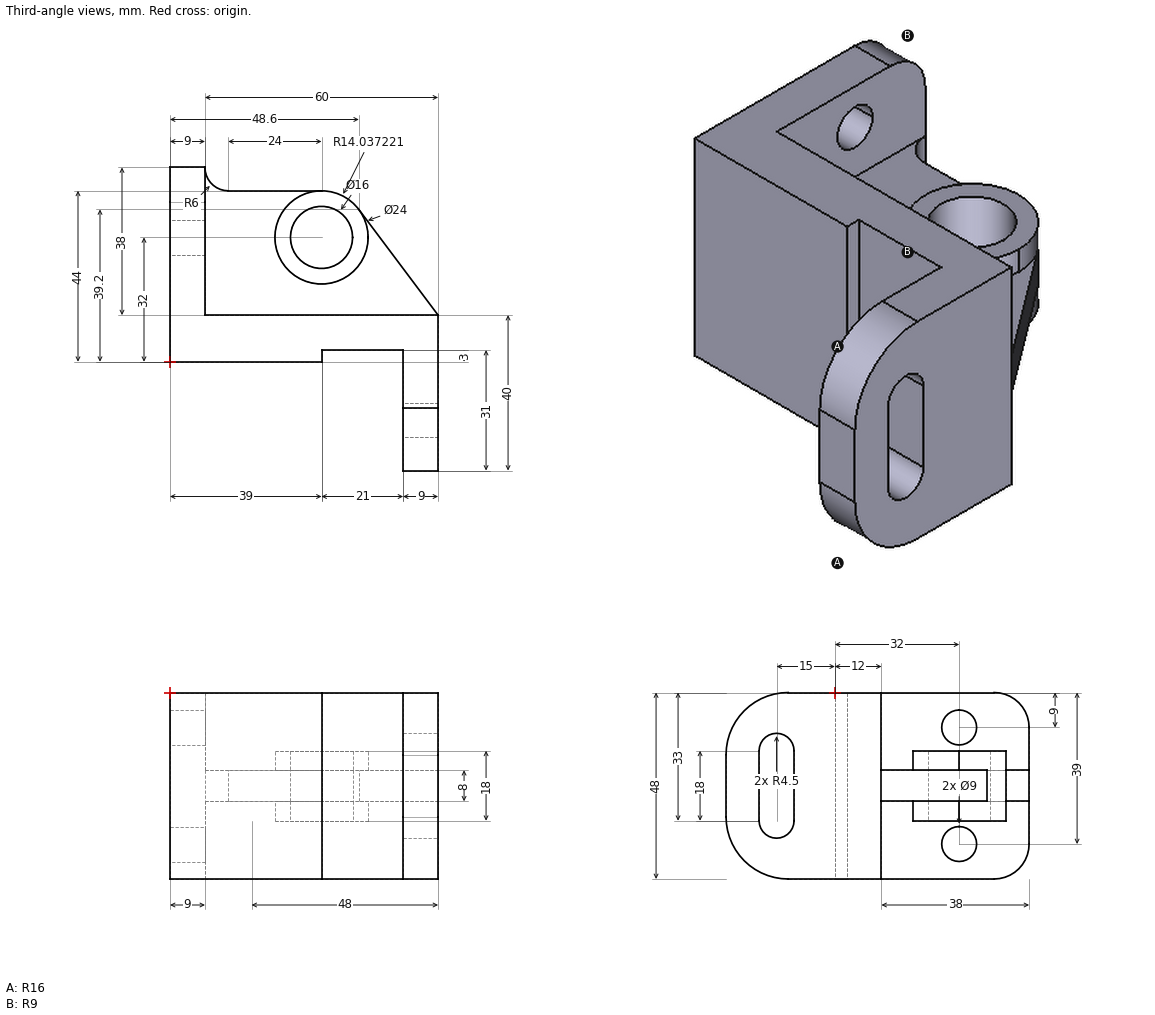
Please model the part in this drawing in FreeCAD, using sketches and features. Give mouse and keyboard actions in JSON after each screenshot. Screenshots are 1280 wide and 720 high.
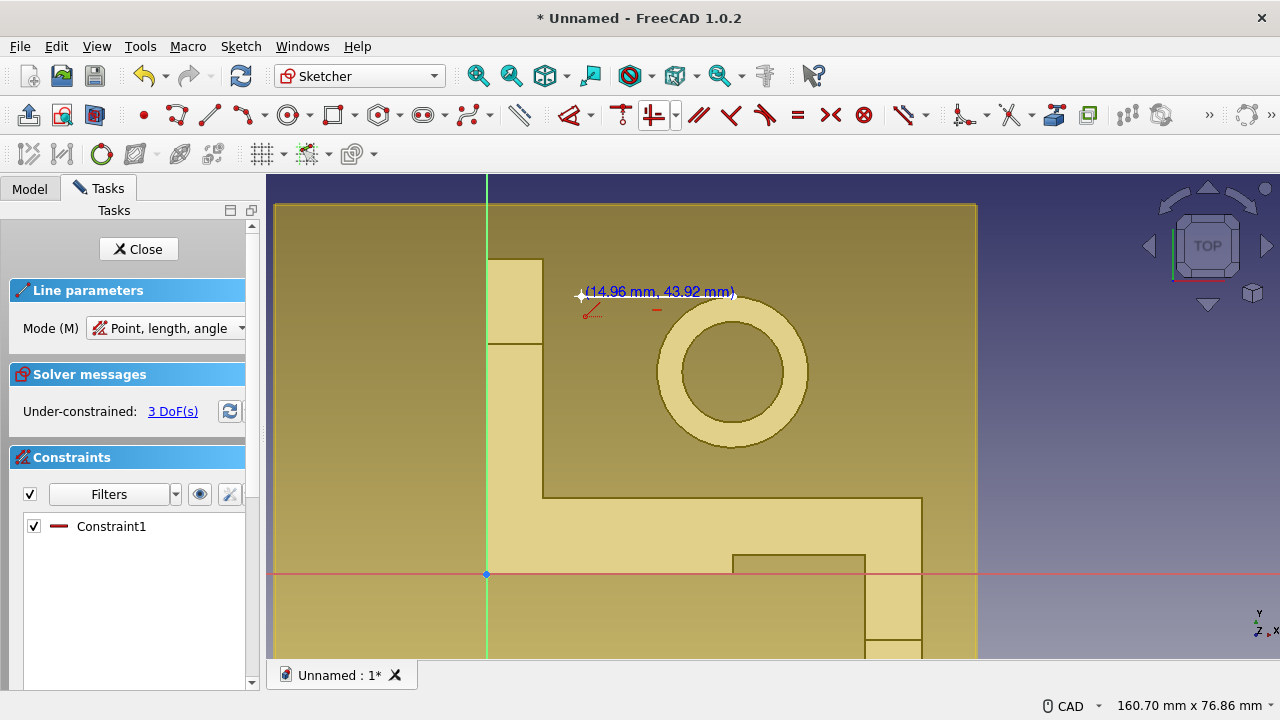
{"action": "left_click", "coordinate": [177, 116]}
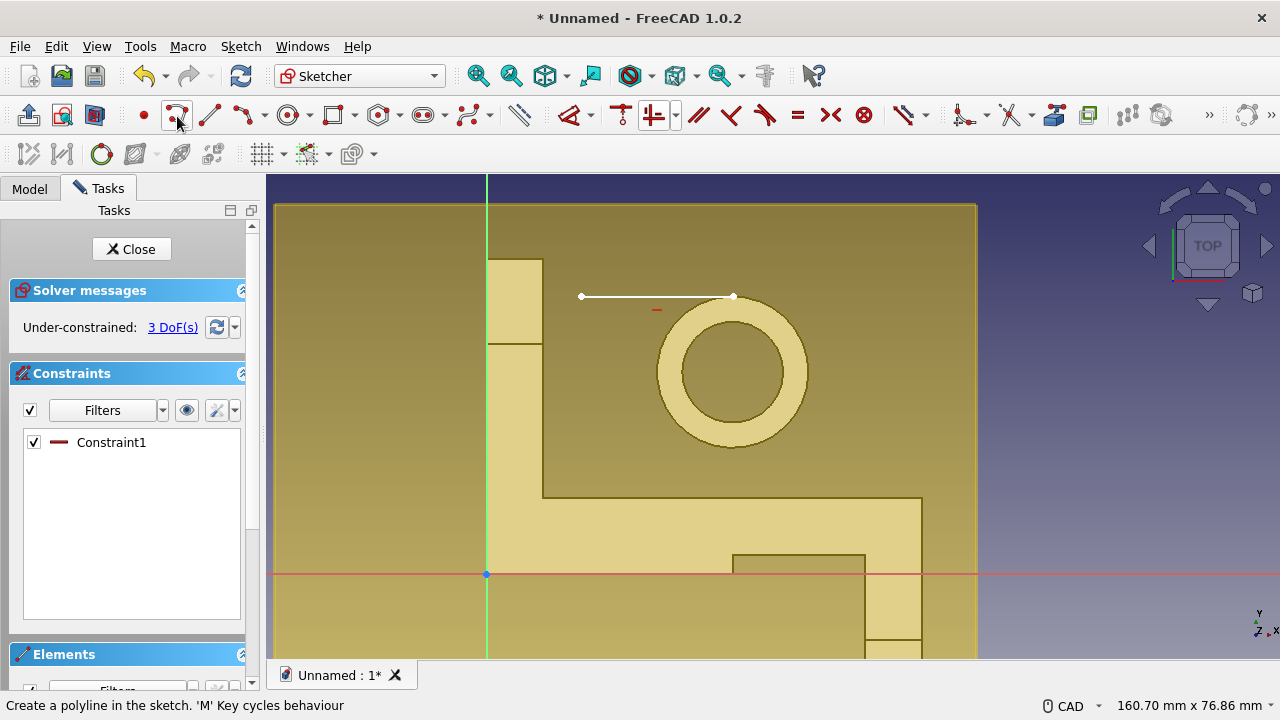
{"action": "left_click", "coordinate": [543, 259]}
{"action": "left_click", "coordinate": [543, 498]}
{"action": "left_click", "coordinate": [922, 498]}
{"action": "left_click", "coordinate": [793, 327]}
{"action": "right_click", "coordinate": [793, 327]}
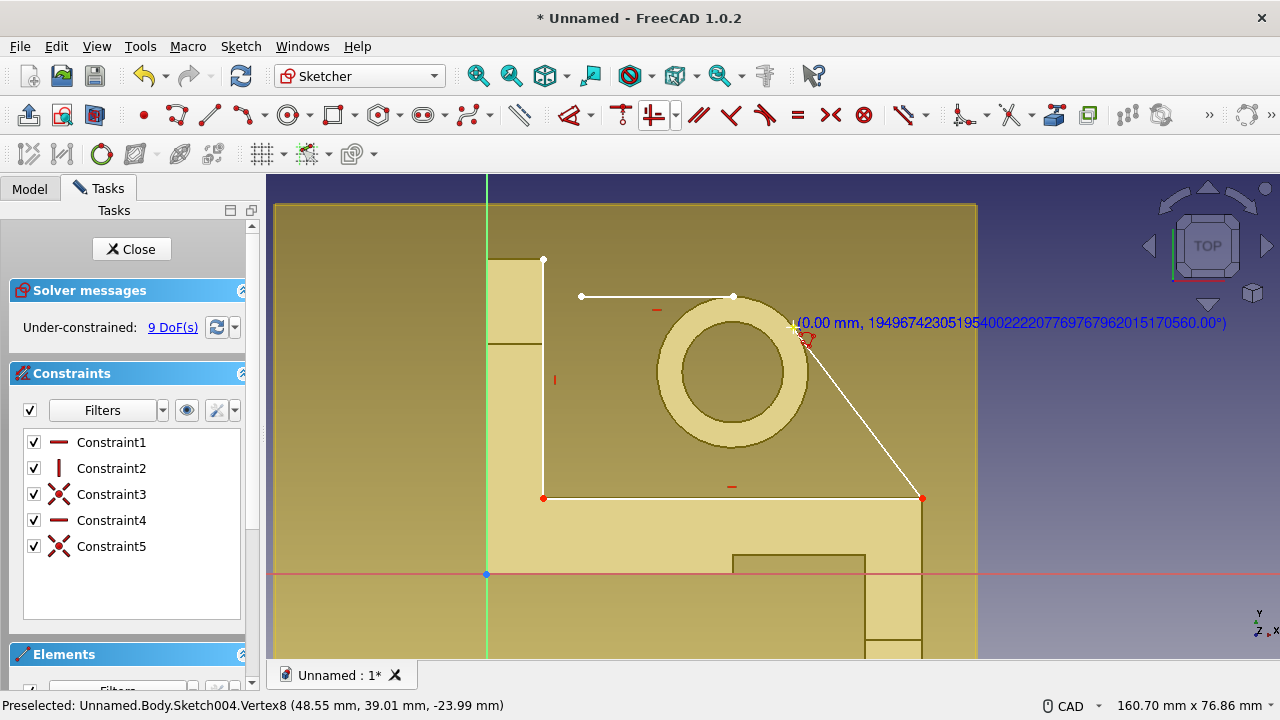
{"action": "key", "text": "g 3 a"}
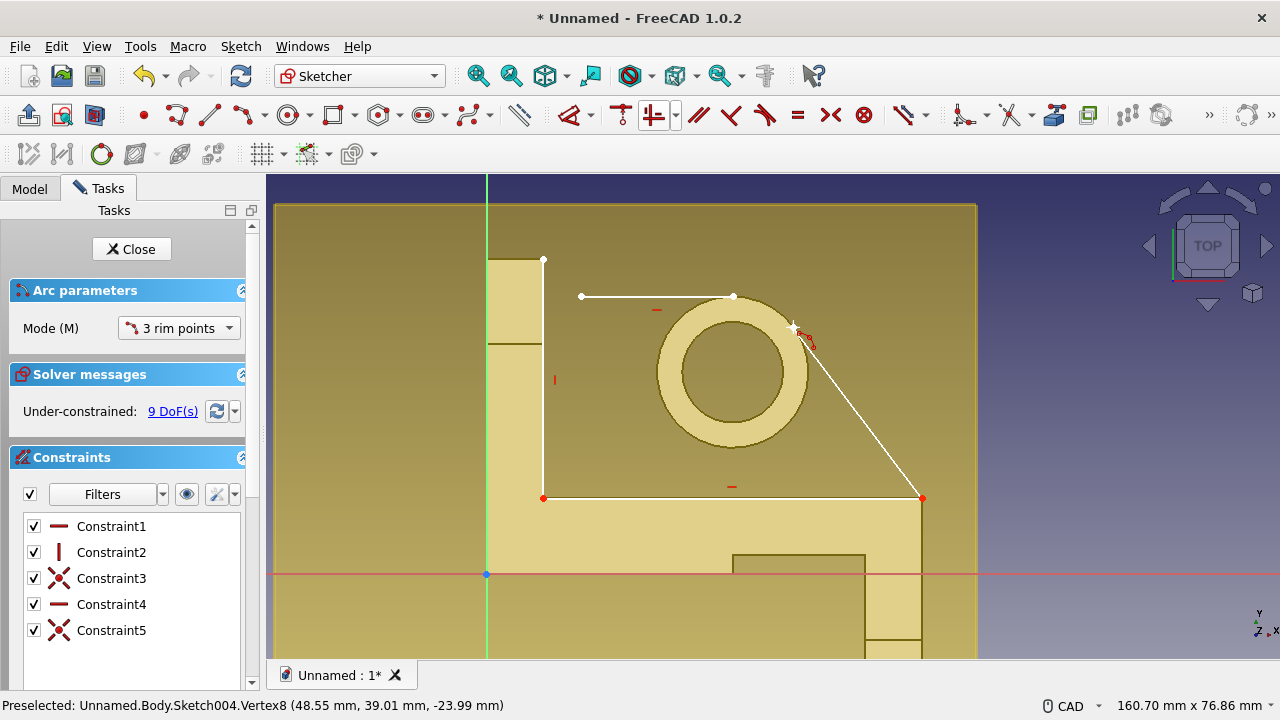
{"action": "left_click", "coordinate": [581, 297]}
{"action": "left_click", "coordinate": [543, 260]}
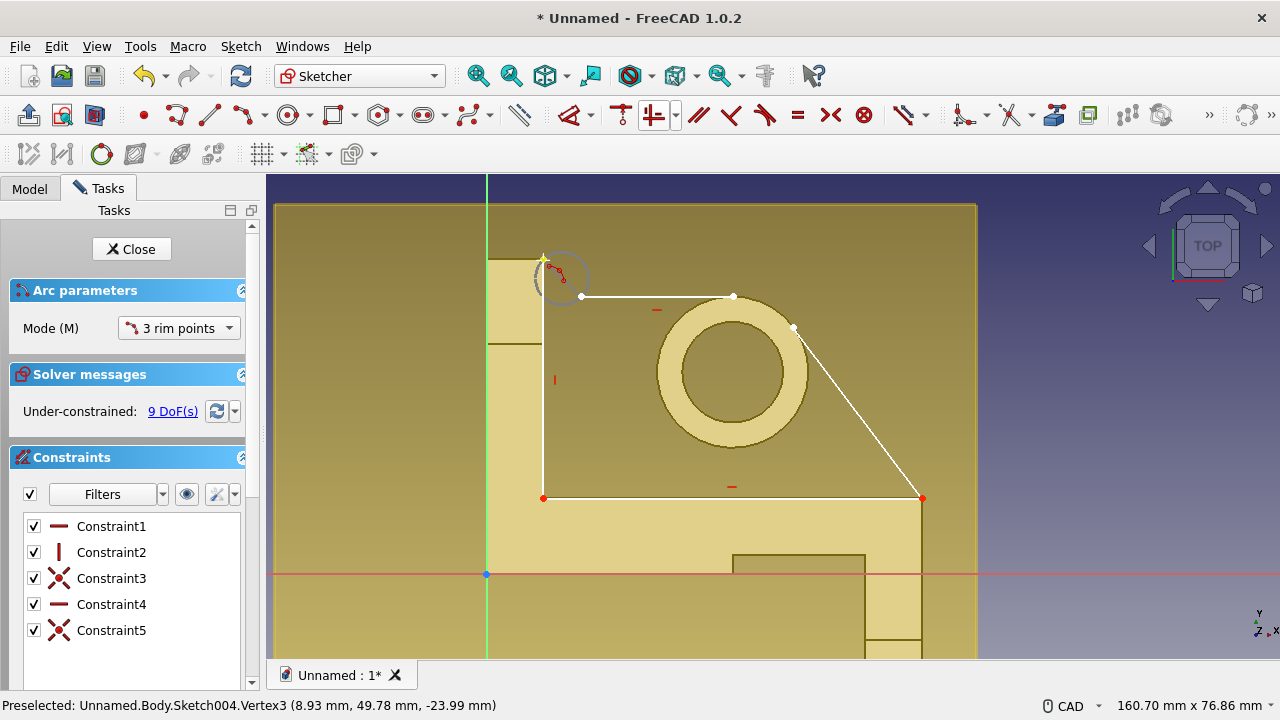
{"action": "scroll", "coordinate": [555, 285], "scroll_direction": "up", "scroll_amount": 2}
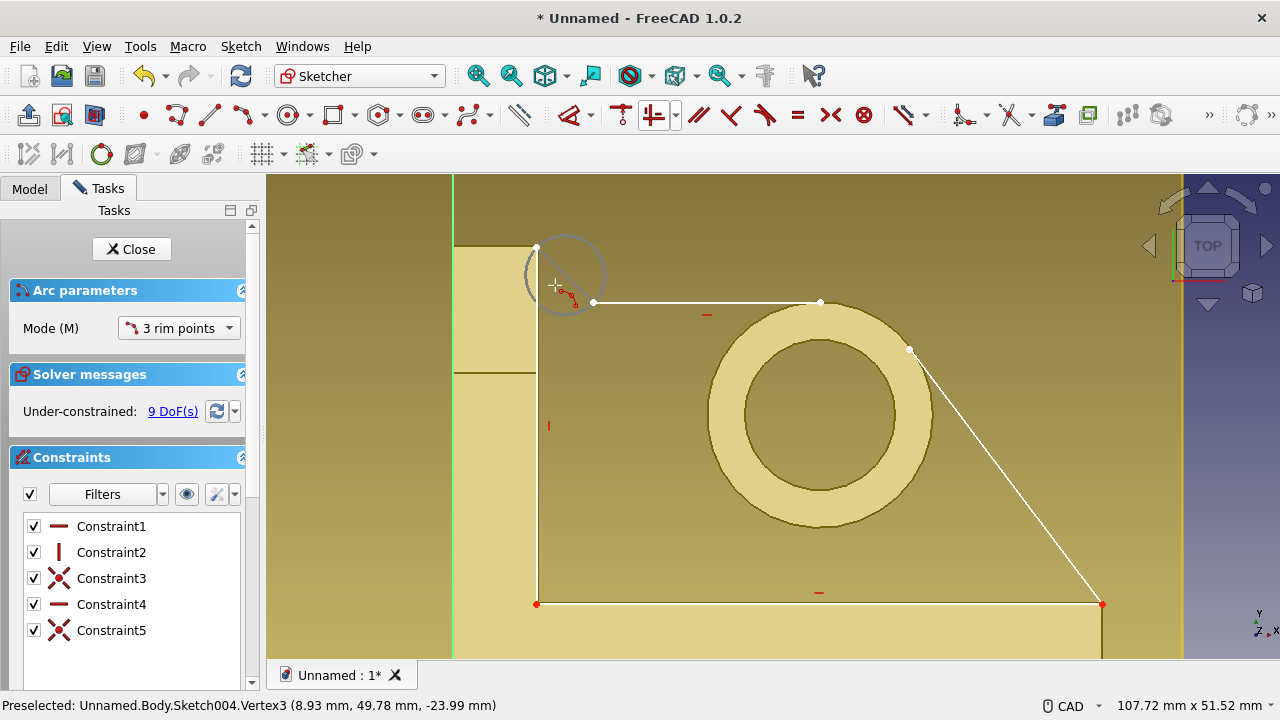
{"action": "left_click", "coordinate": [554, 285]}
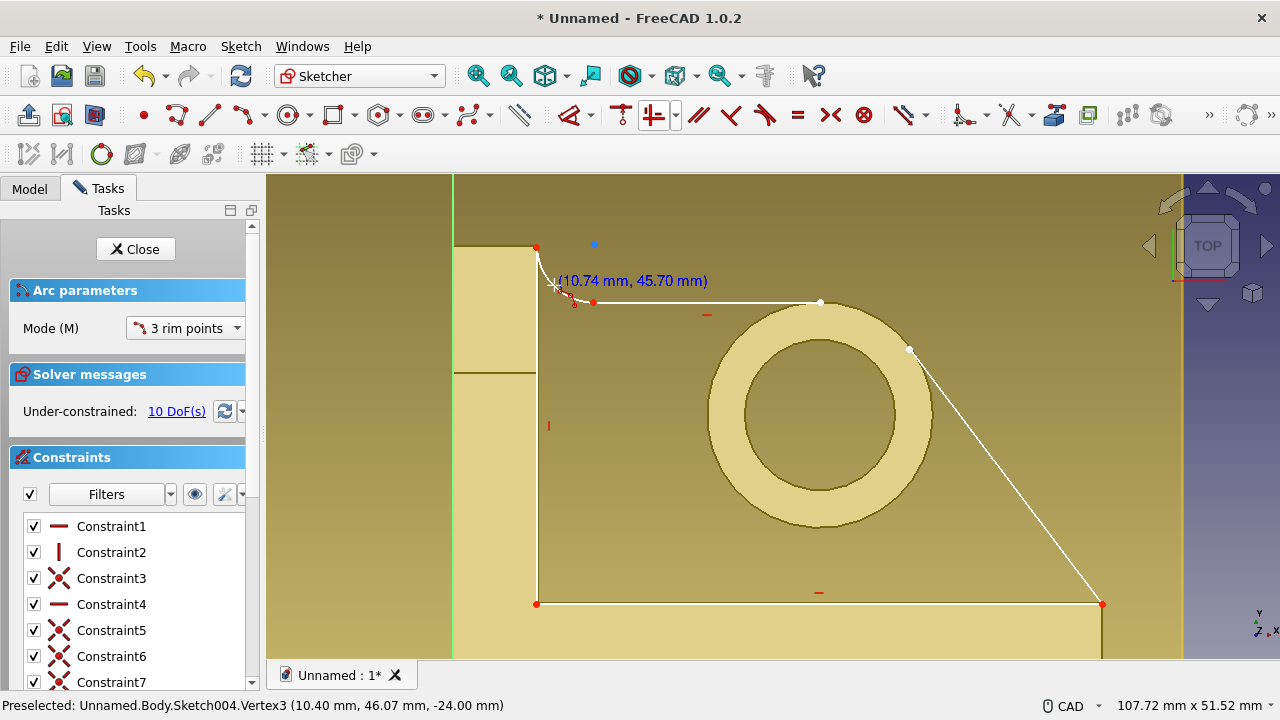
{"action": "left_click", "coordinate": [910, 349]}
{"action": "left_click", "coordinate": [820, 303]}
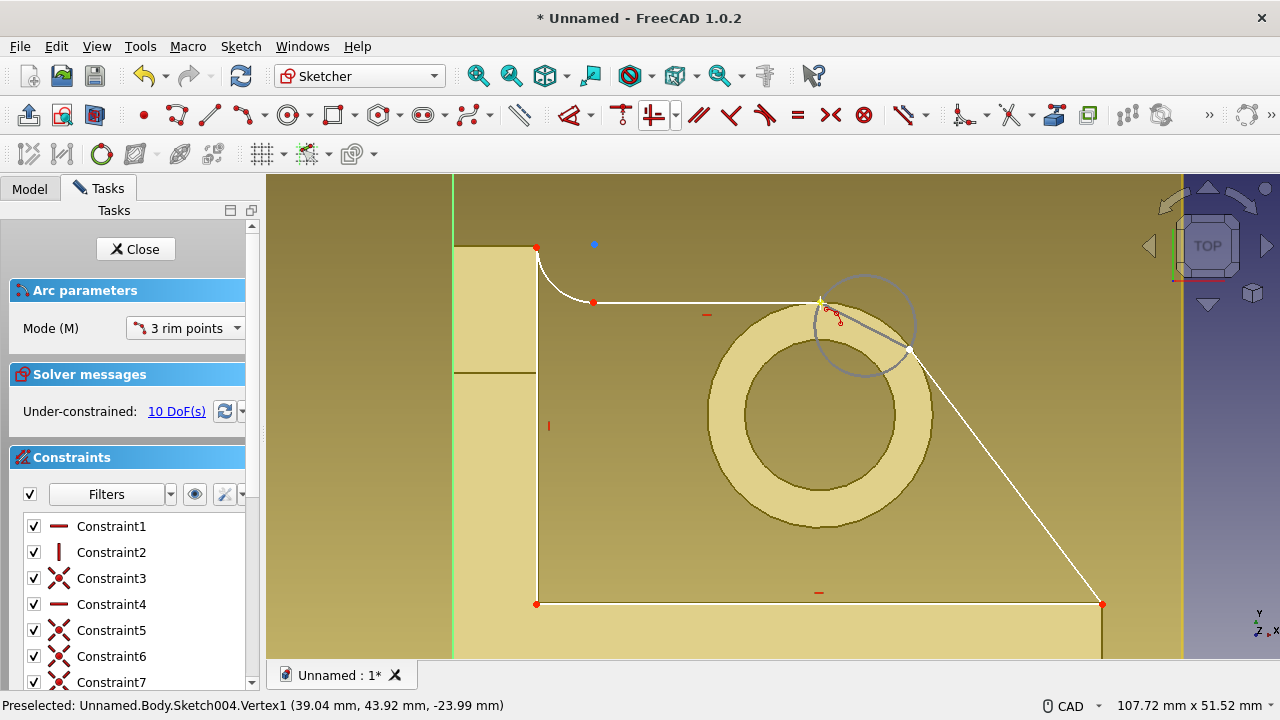
{"action": "scroll", "coordinate": [870, 316], "scroll_direction": "up", "scroll_amount": 3}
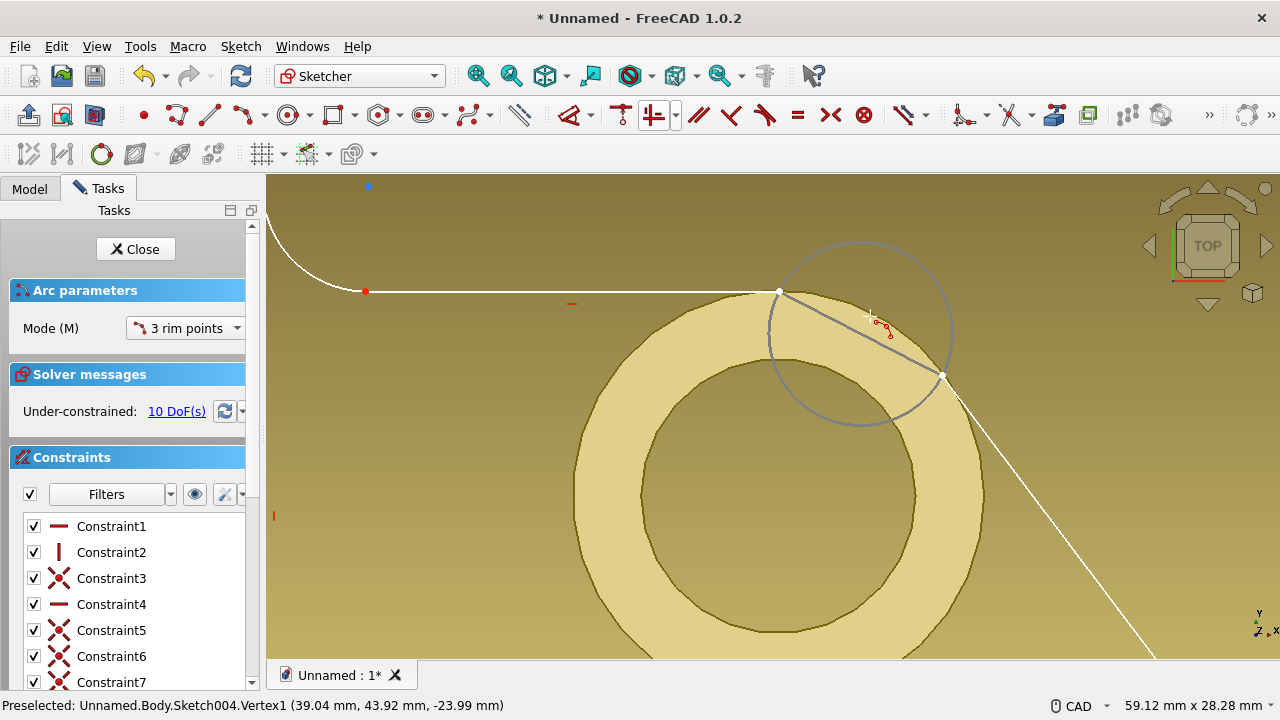
{"action": "left_click", "coordinate": [869, 315]}
{"action": "key", "text": "Escape"}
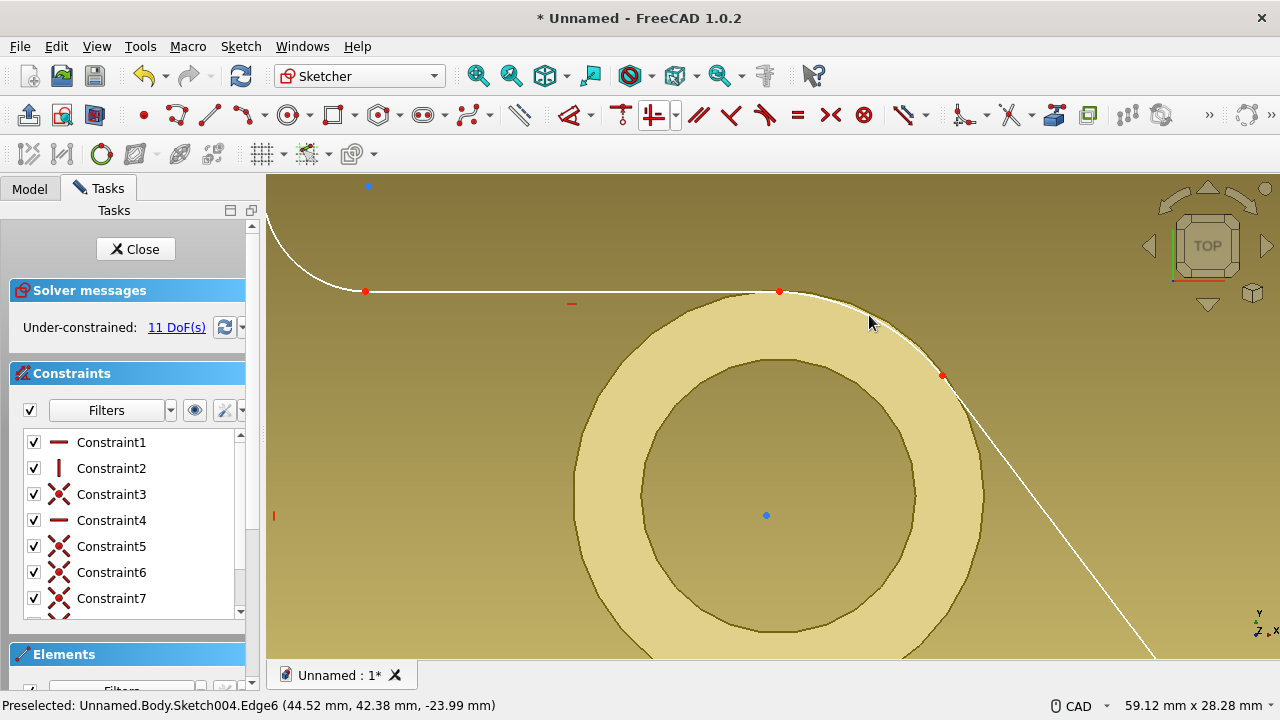
{"action": "left_click", "coordinate": [655, 292]}